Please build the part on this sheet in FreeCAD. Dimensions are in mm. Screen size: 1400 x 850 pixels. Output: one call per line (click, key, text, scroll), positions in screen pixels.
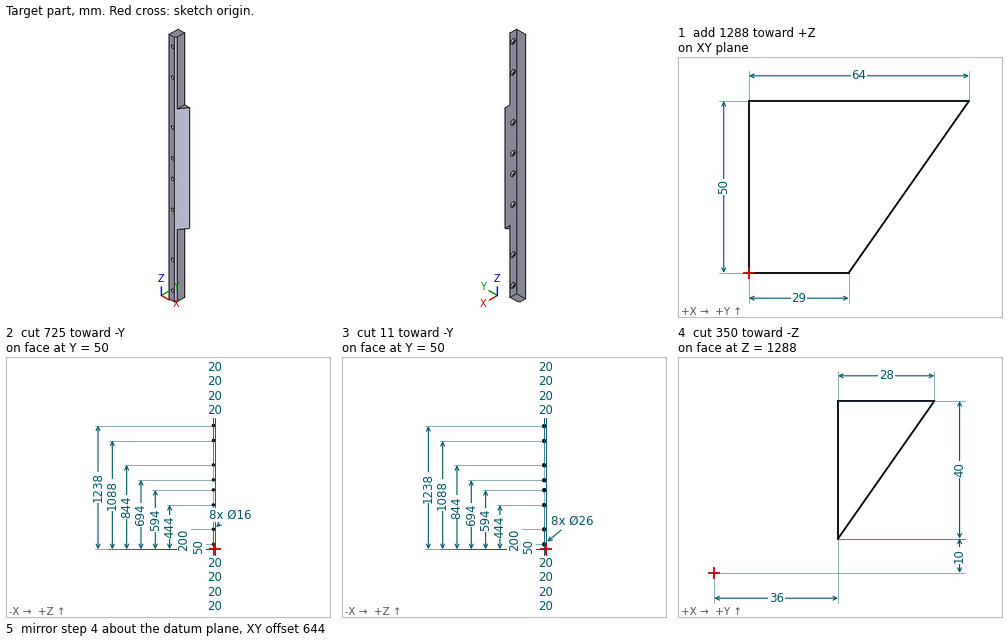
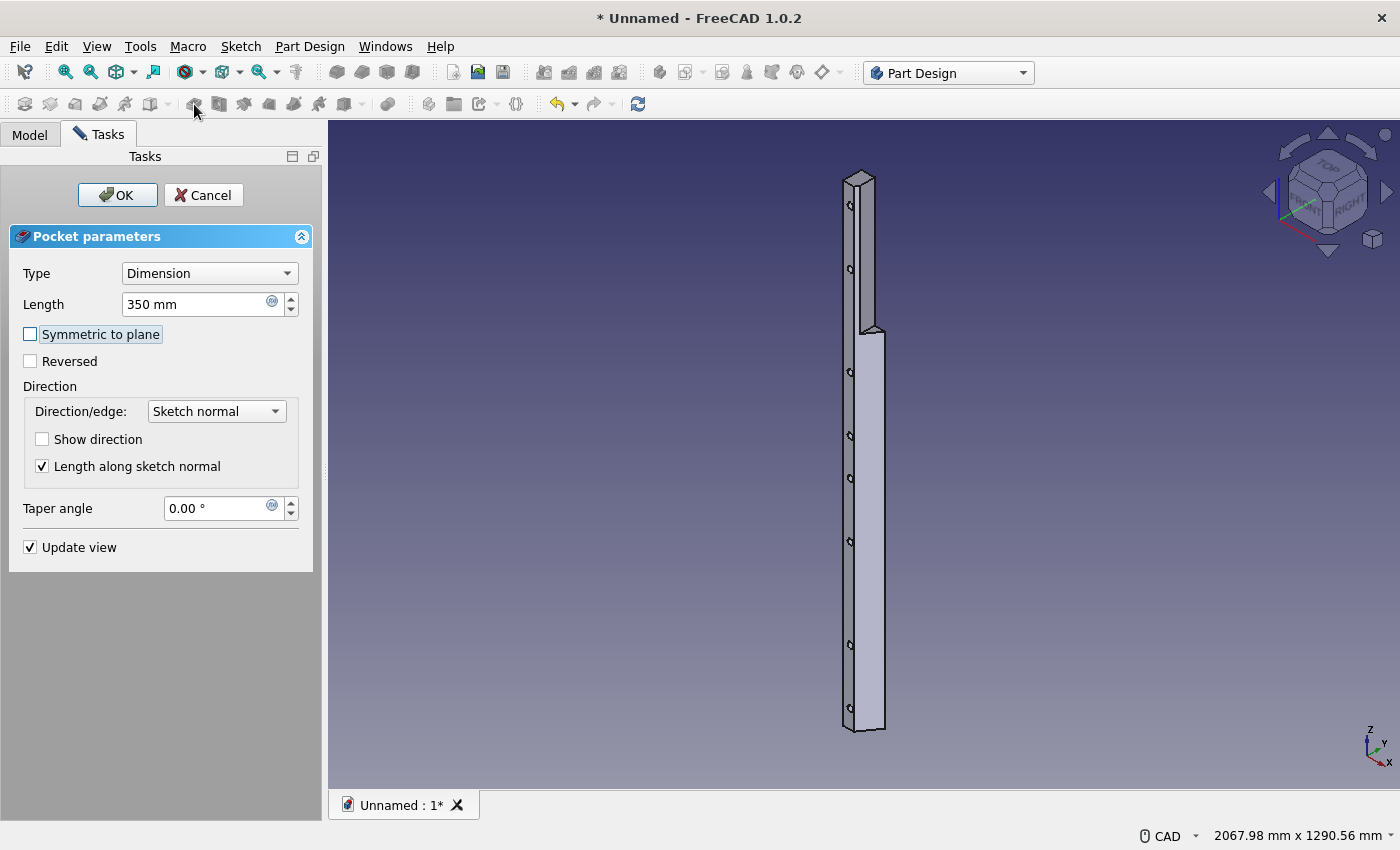
click(118, 195)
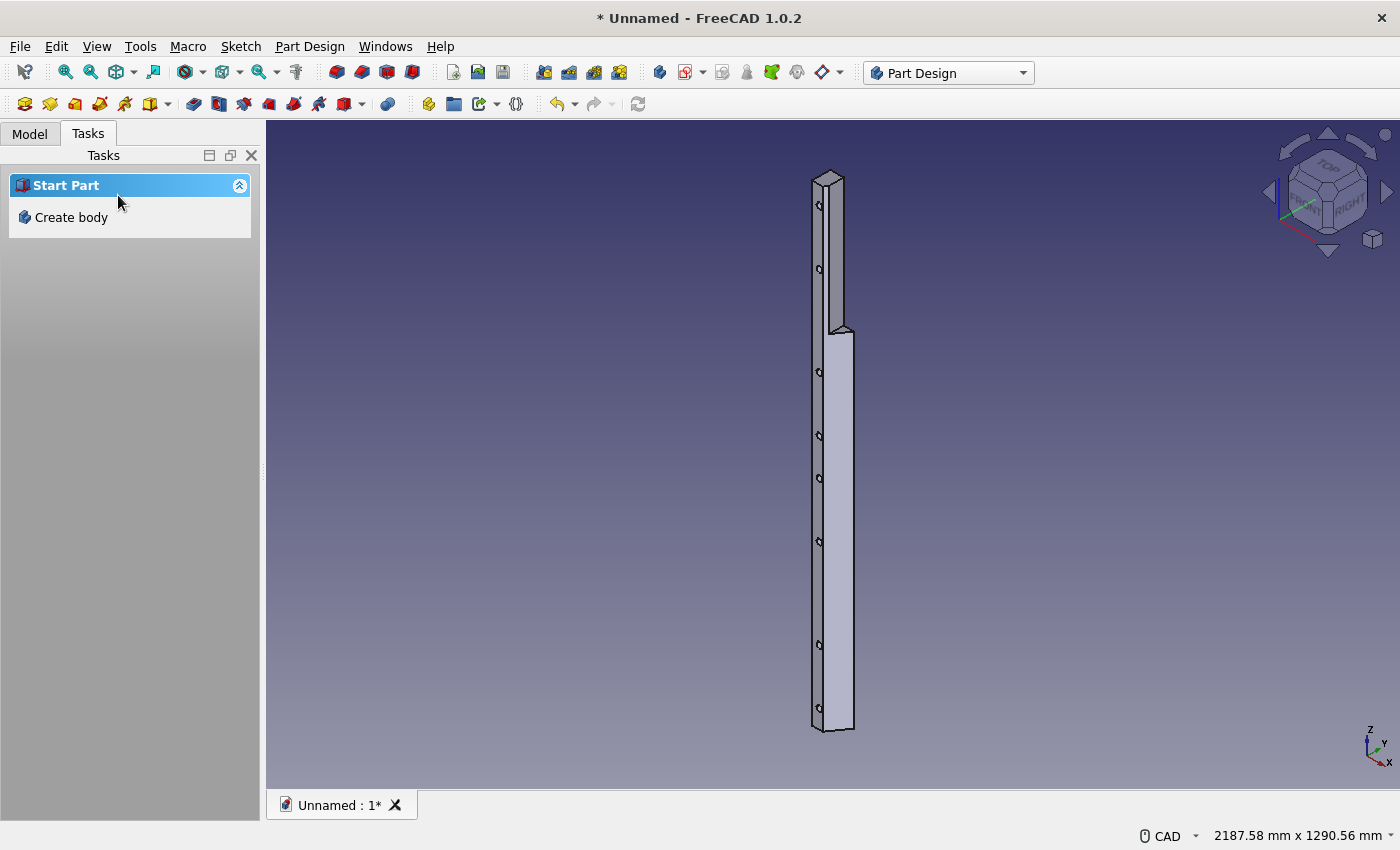
click(30, 134)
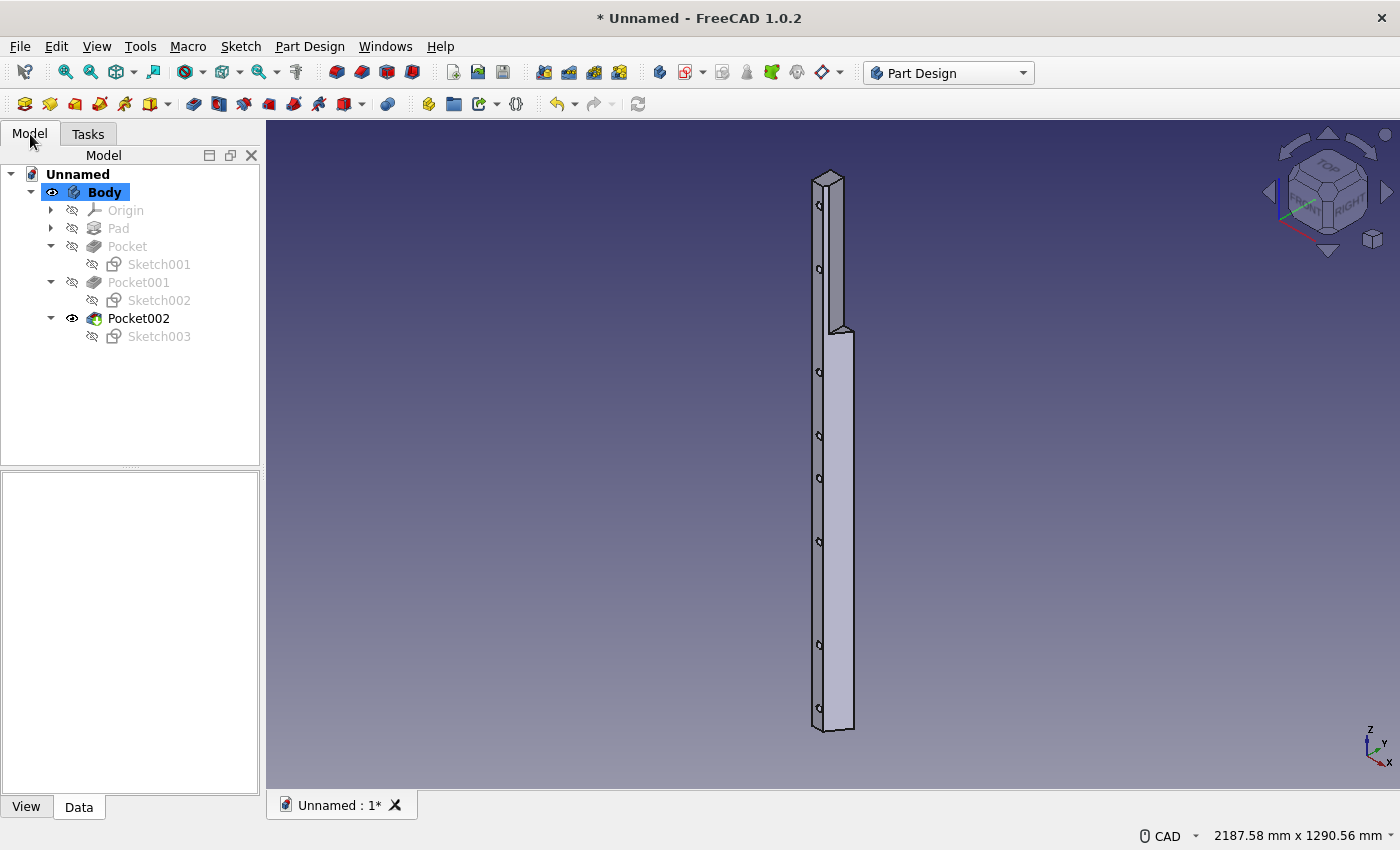
click(51, 210)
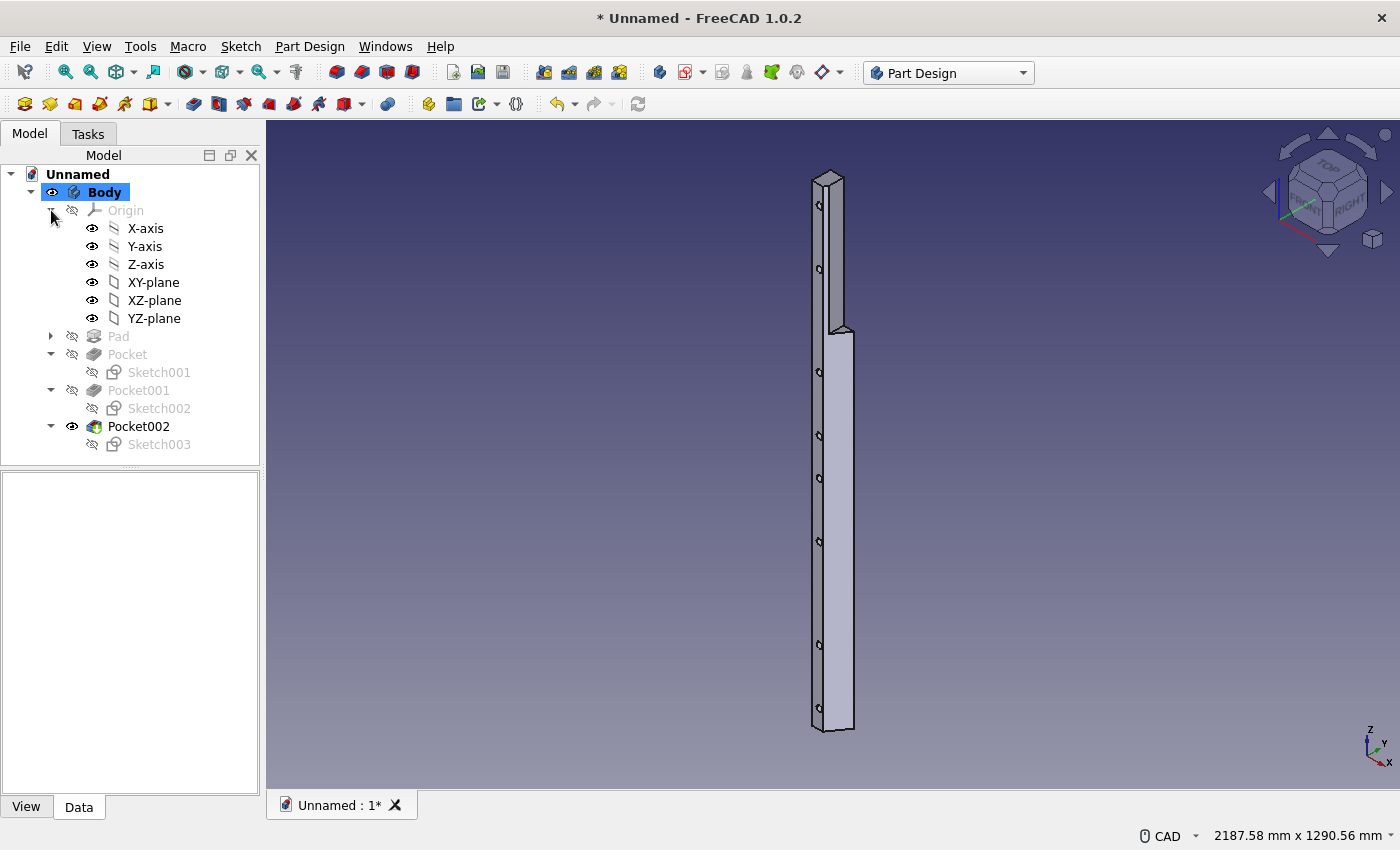
click(137, 282)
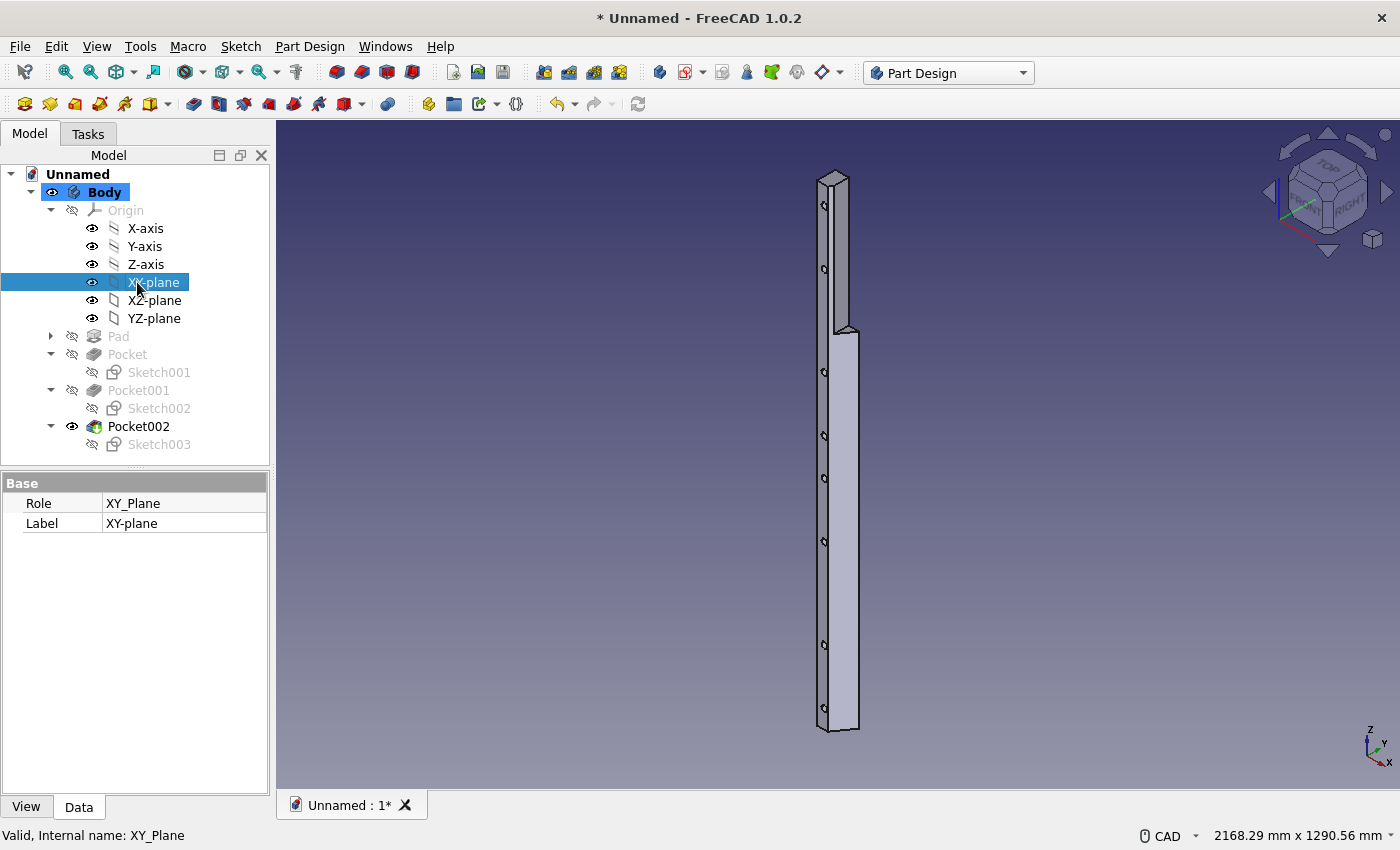
click(822, 72)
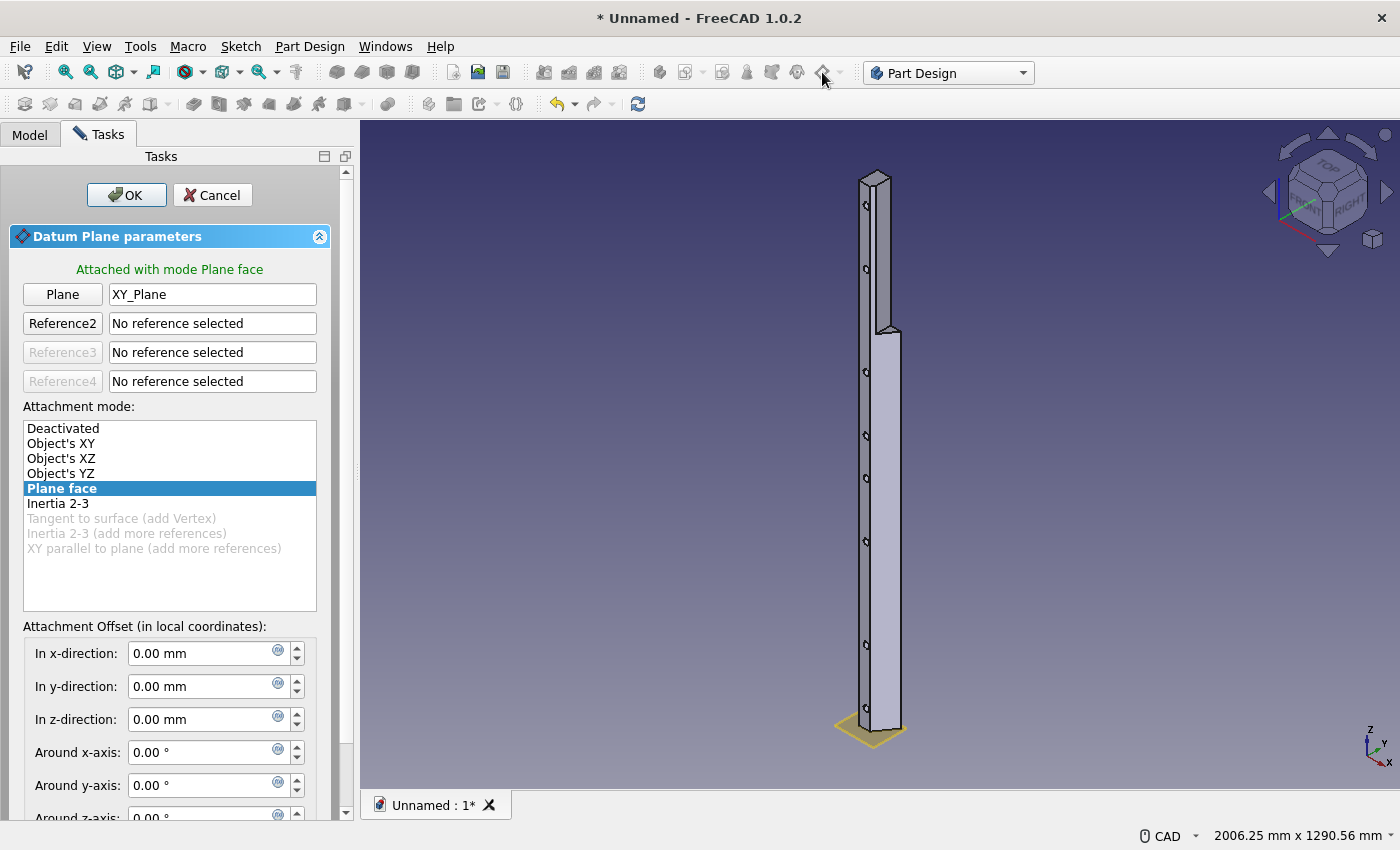
triple_click(210, 720)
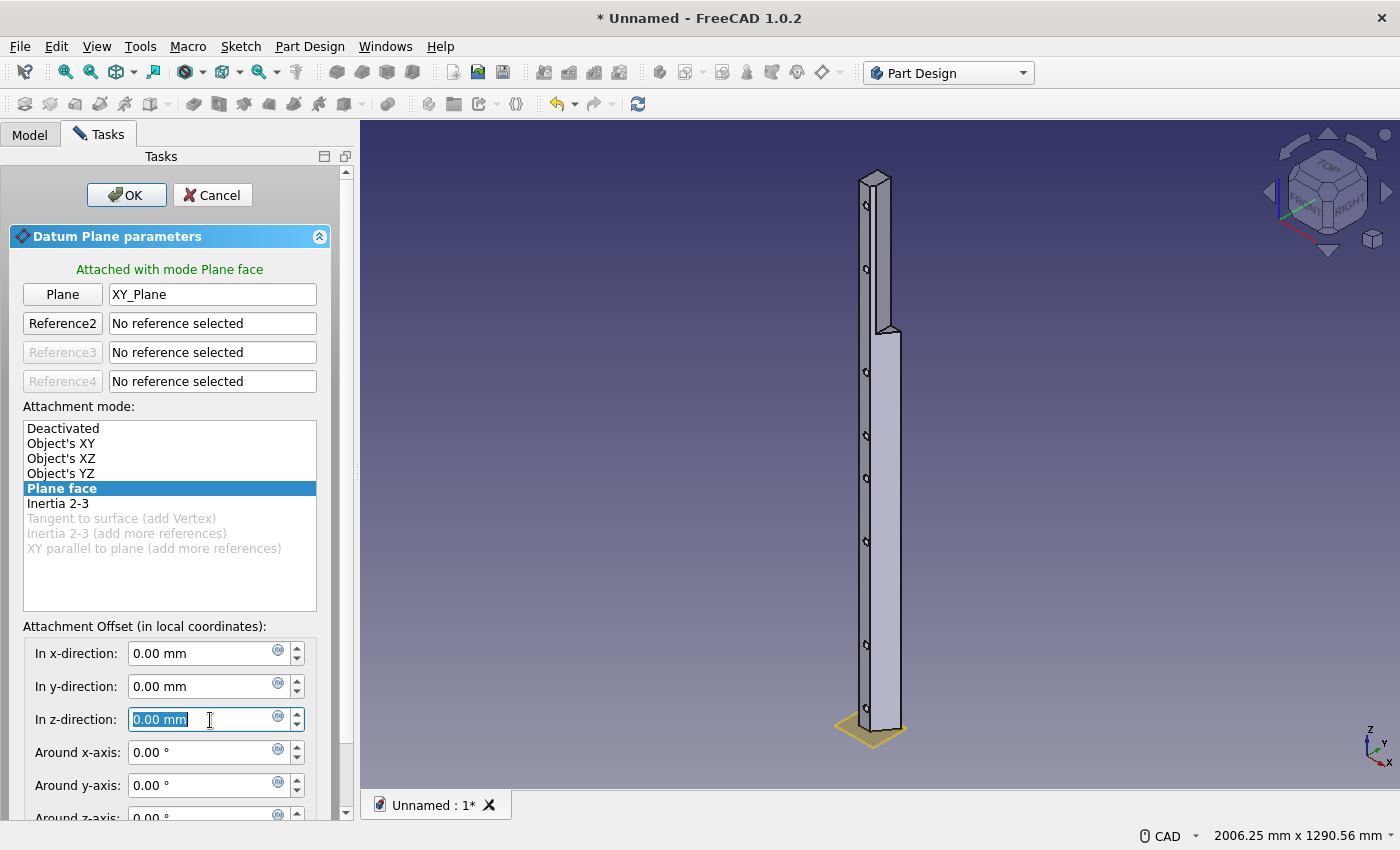
text(644)
key(Tab)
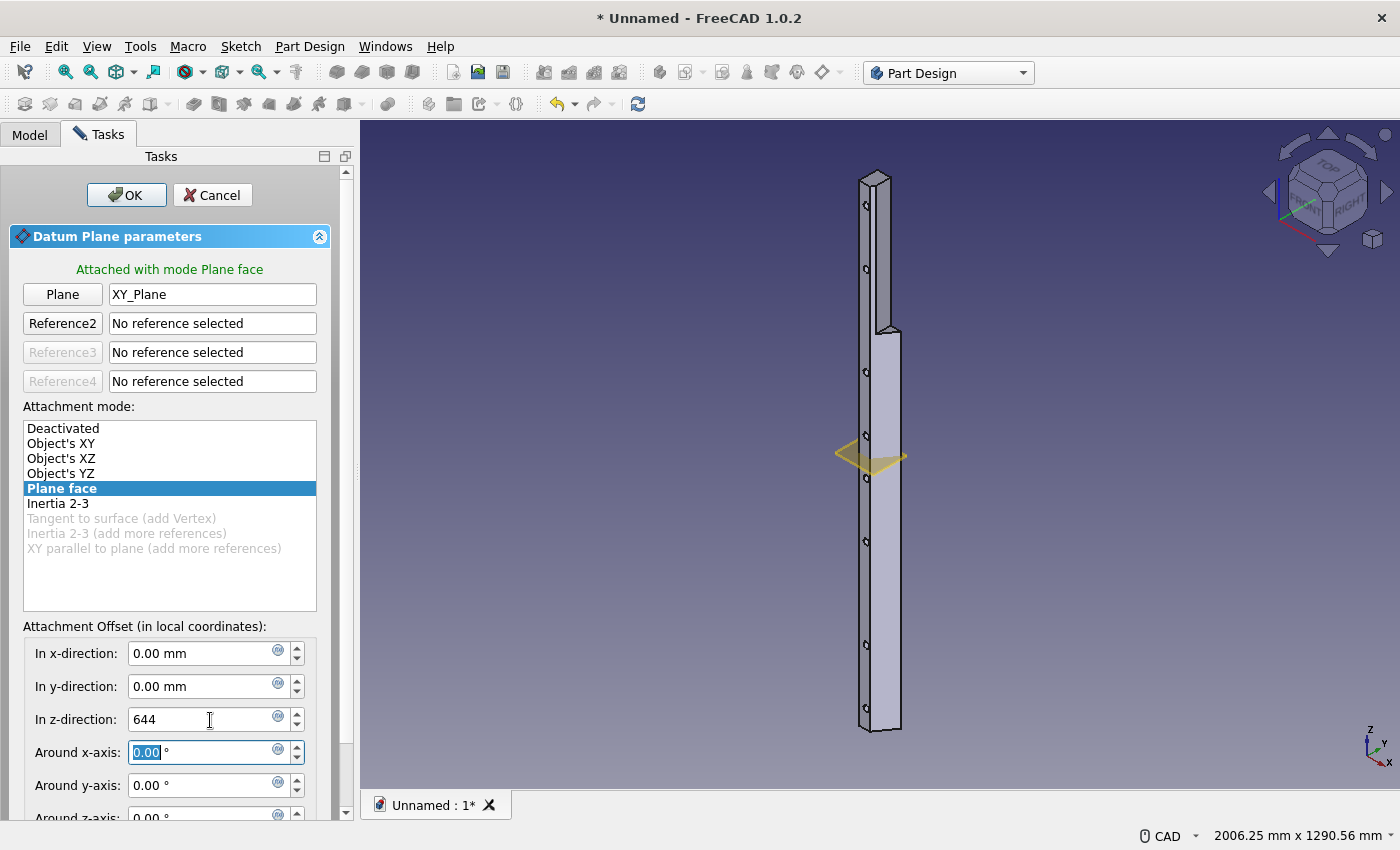
click(127, 195)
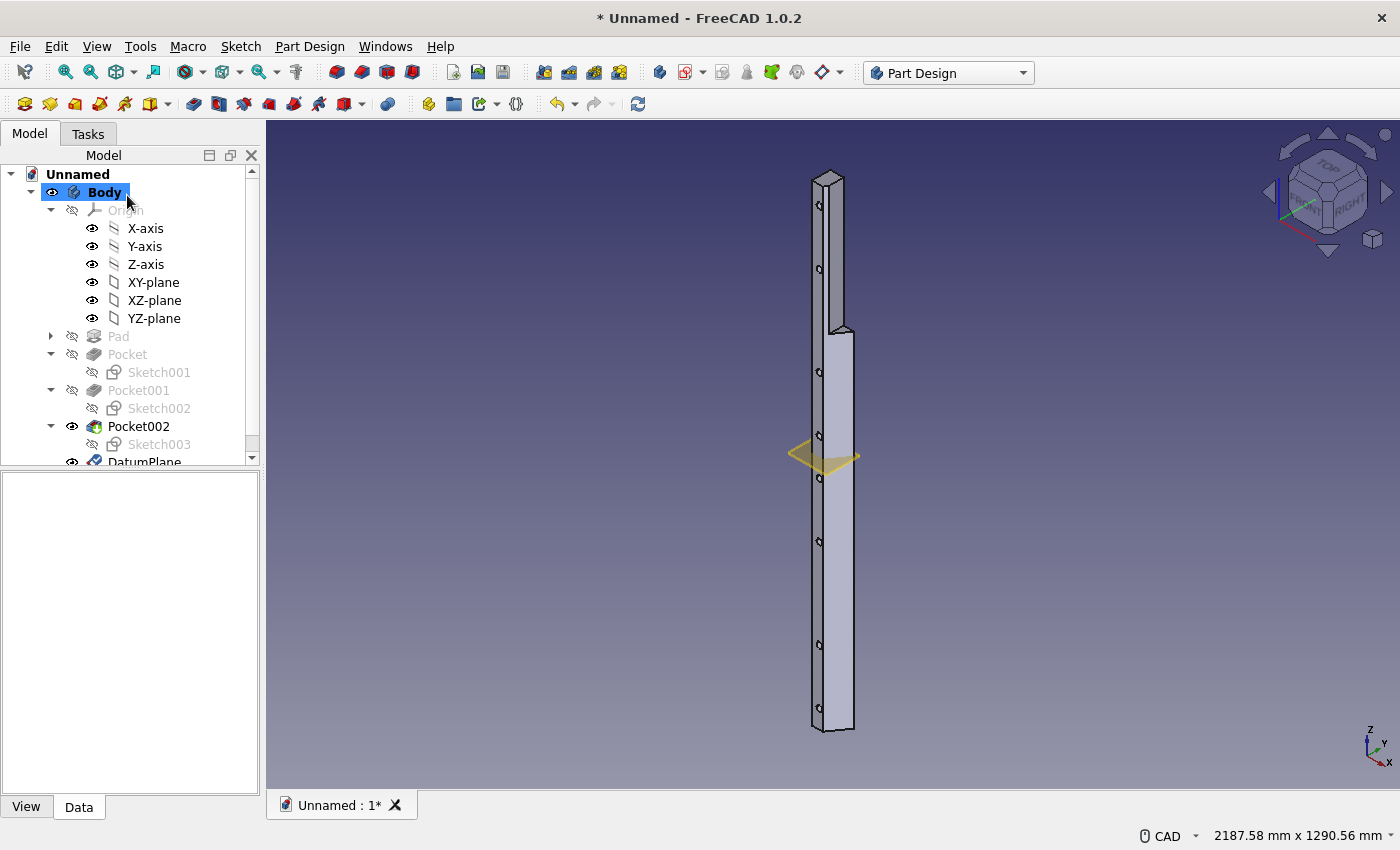
click(117, 426)